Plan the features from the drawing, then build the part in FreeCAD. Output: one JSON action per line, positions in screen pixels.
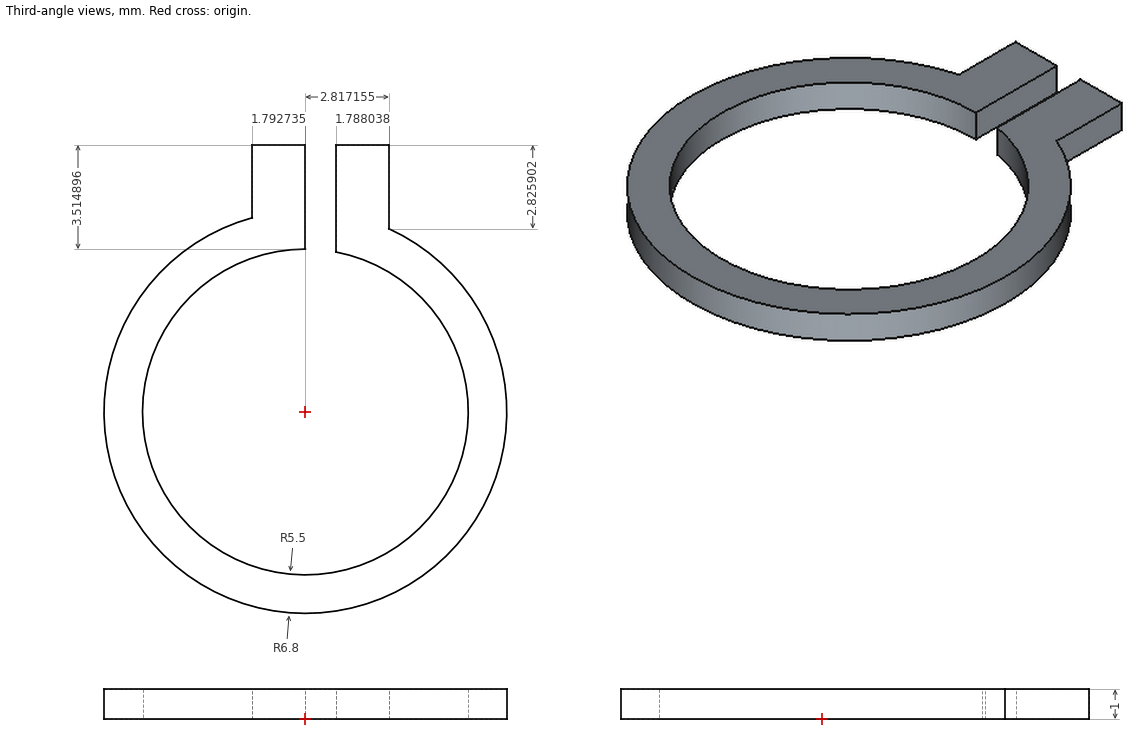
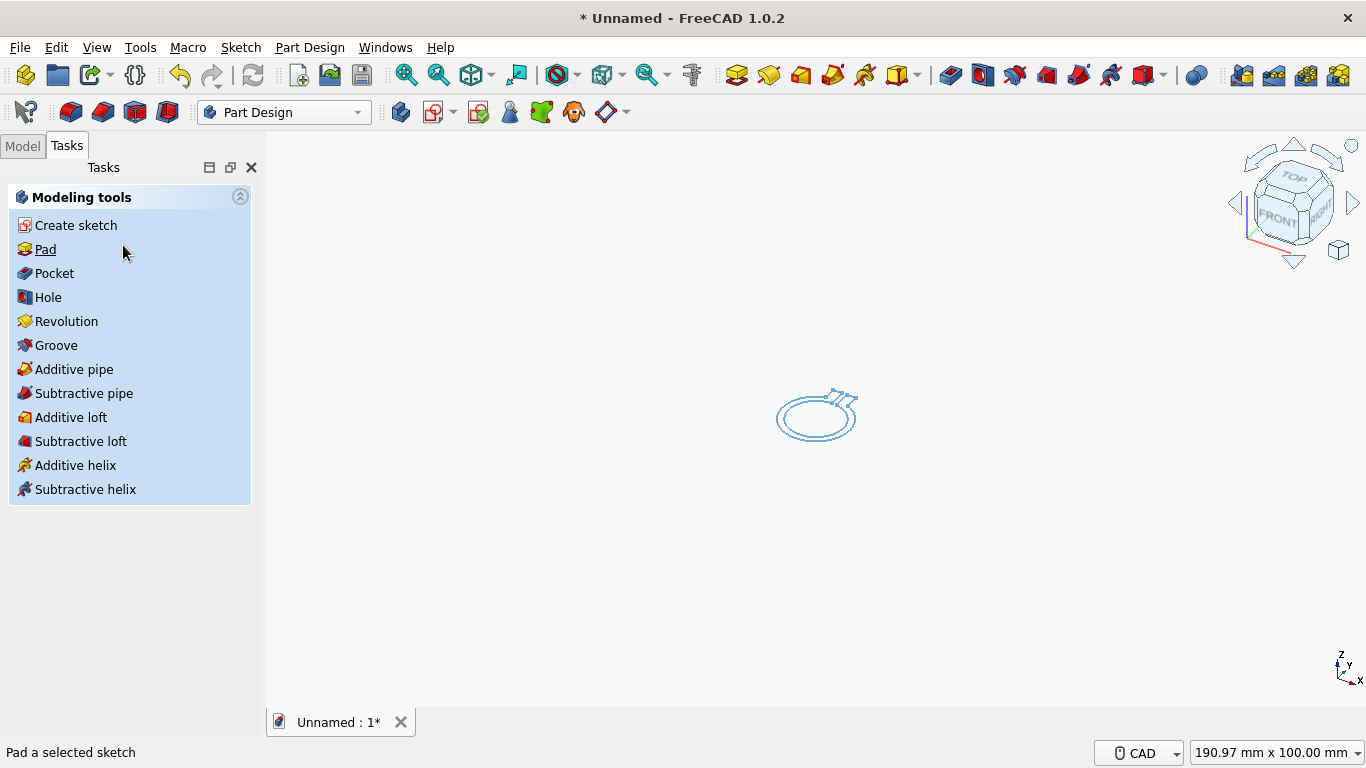
{"action": "left_click", "coordinate": [738, 76]}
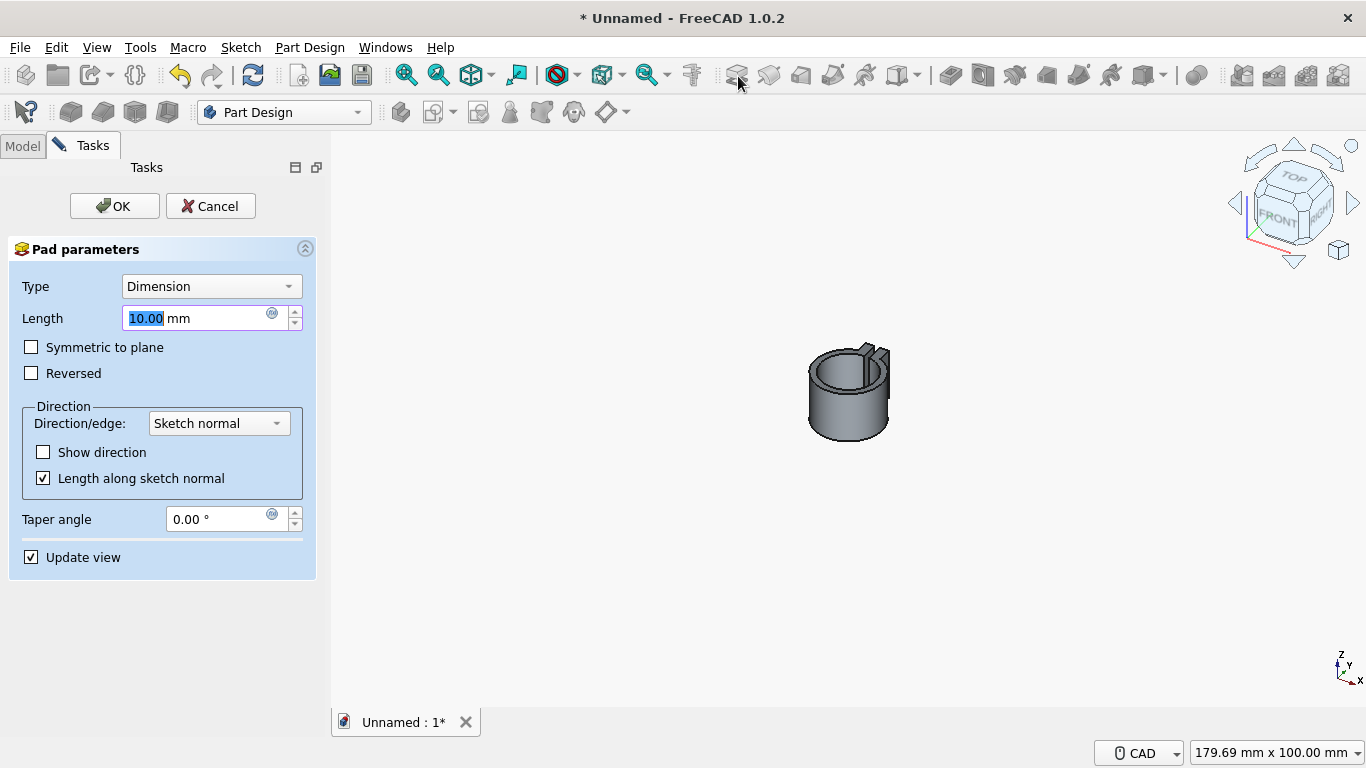
{"action": "type", "text": "1"}
{"action": "key", "text": "Tab"}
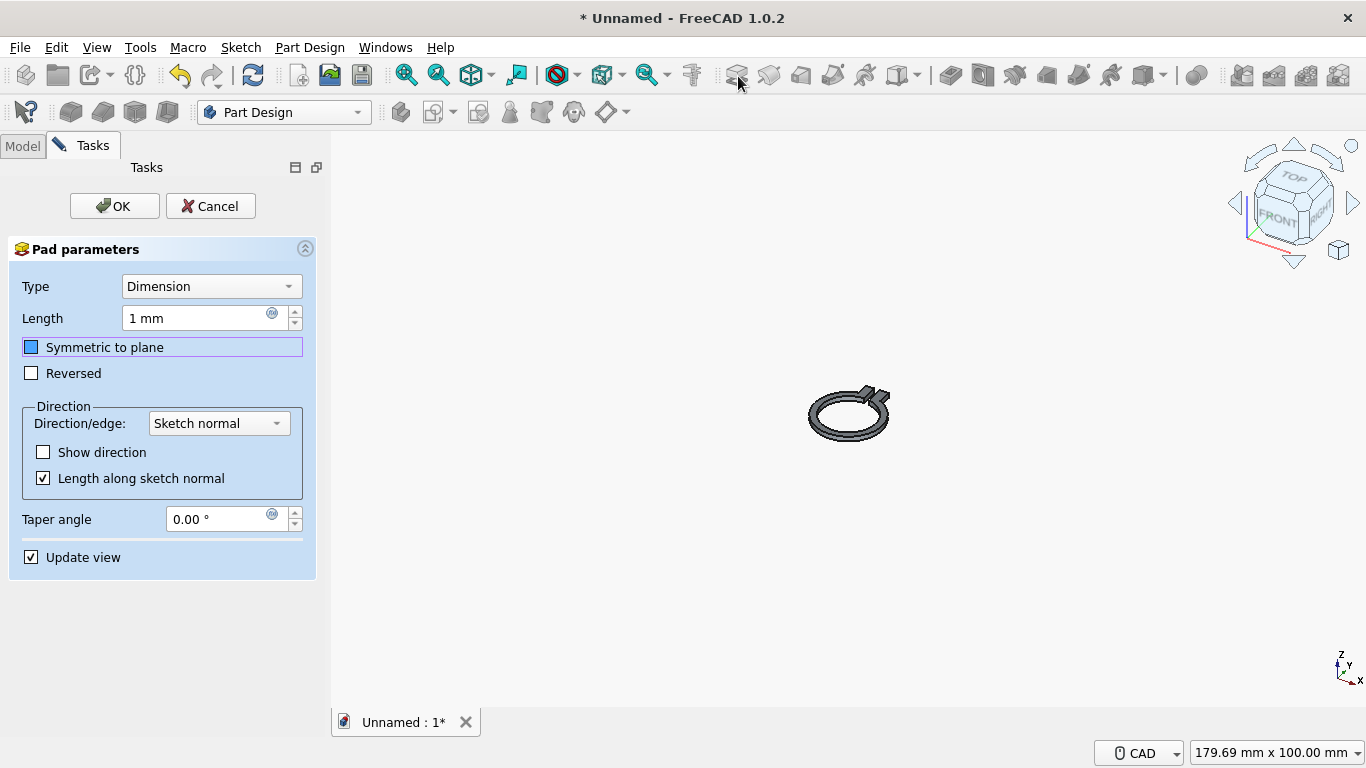
{"action": "left_click", "coordinate": [115, 206]}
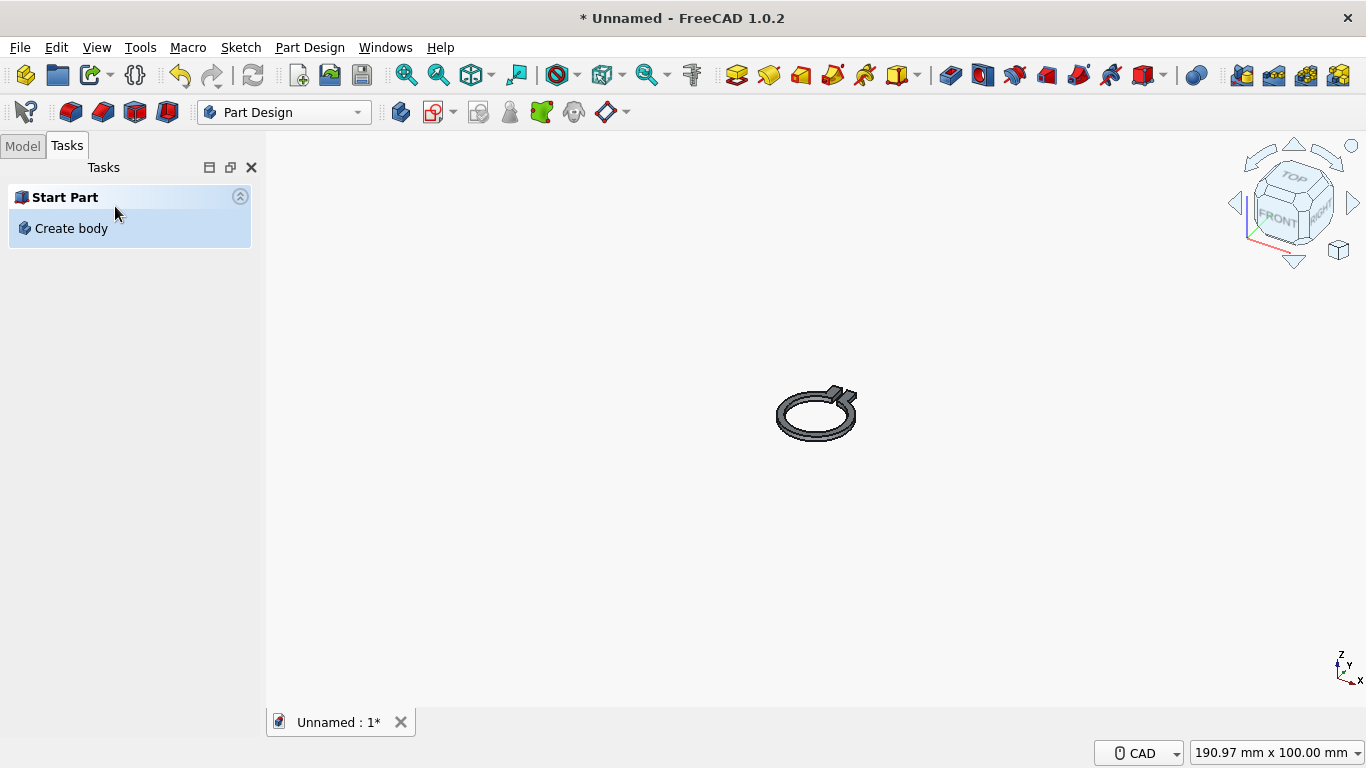
{"action": "key", "text": "0"}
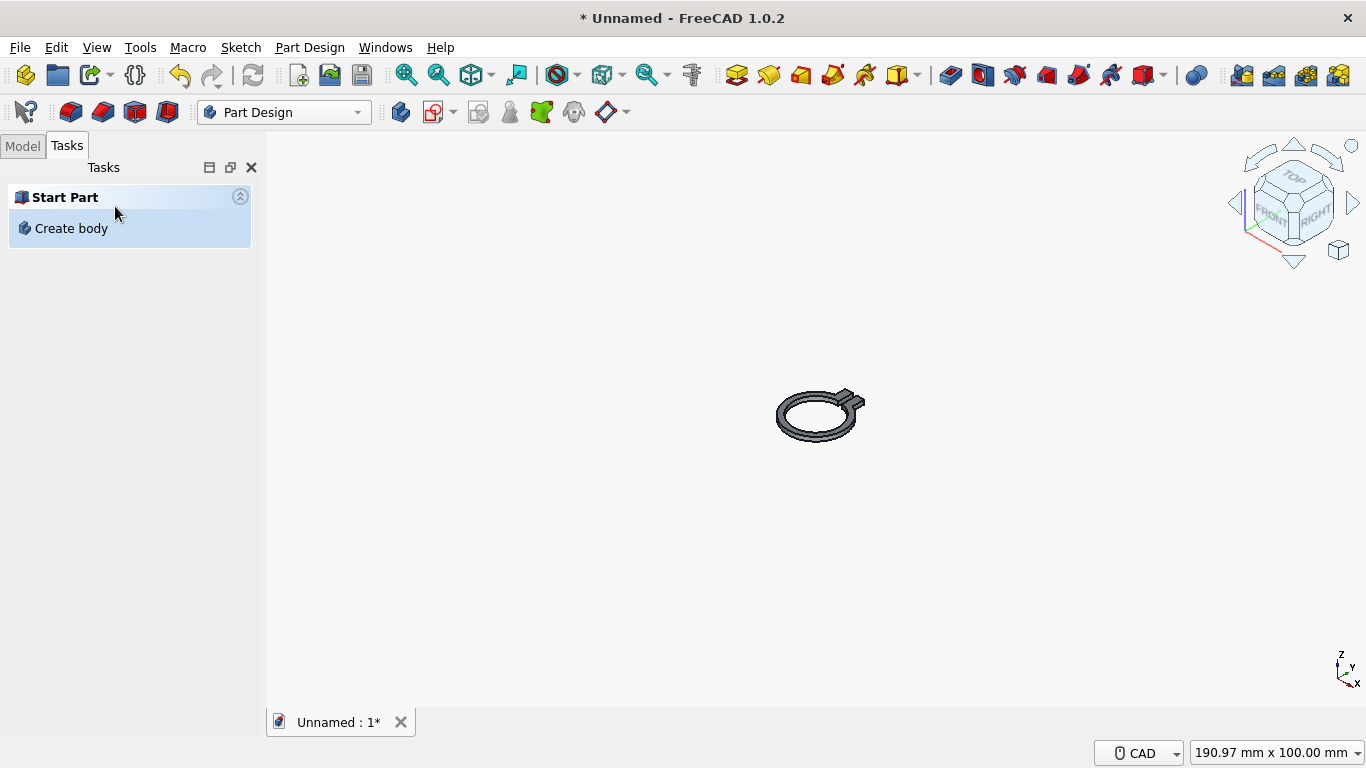
{"action": "left_click", "coordinate": [408, 76]}